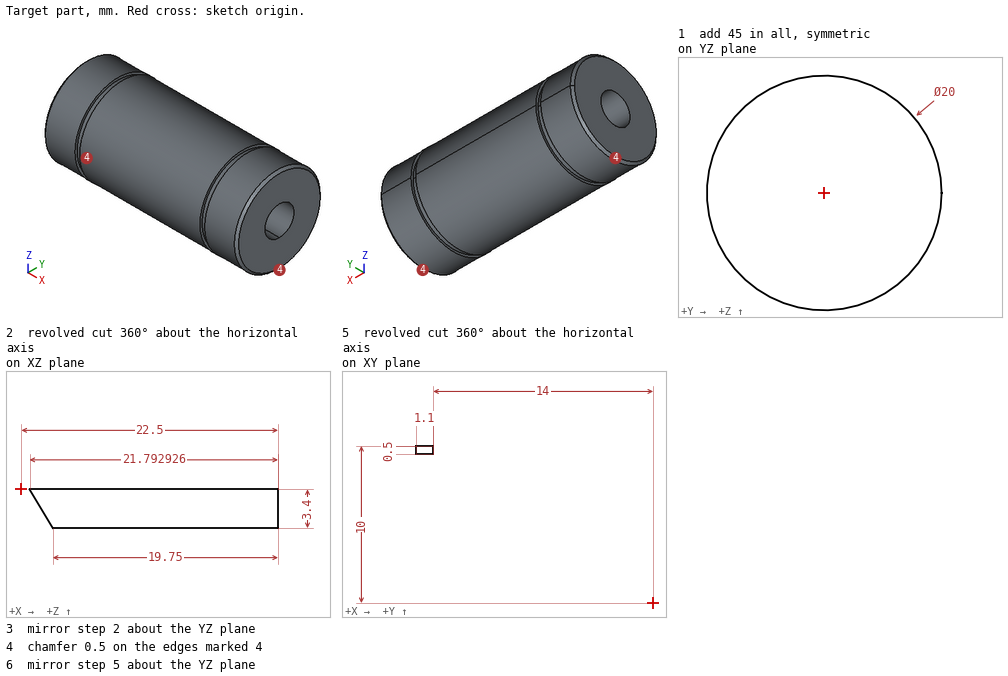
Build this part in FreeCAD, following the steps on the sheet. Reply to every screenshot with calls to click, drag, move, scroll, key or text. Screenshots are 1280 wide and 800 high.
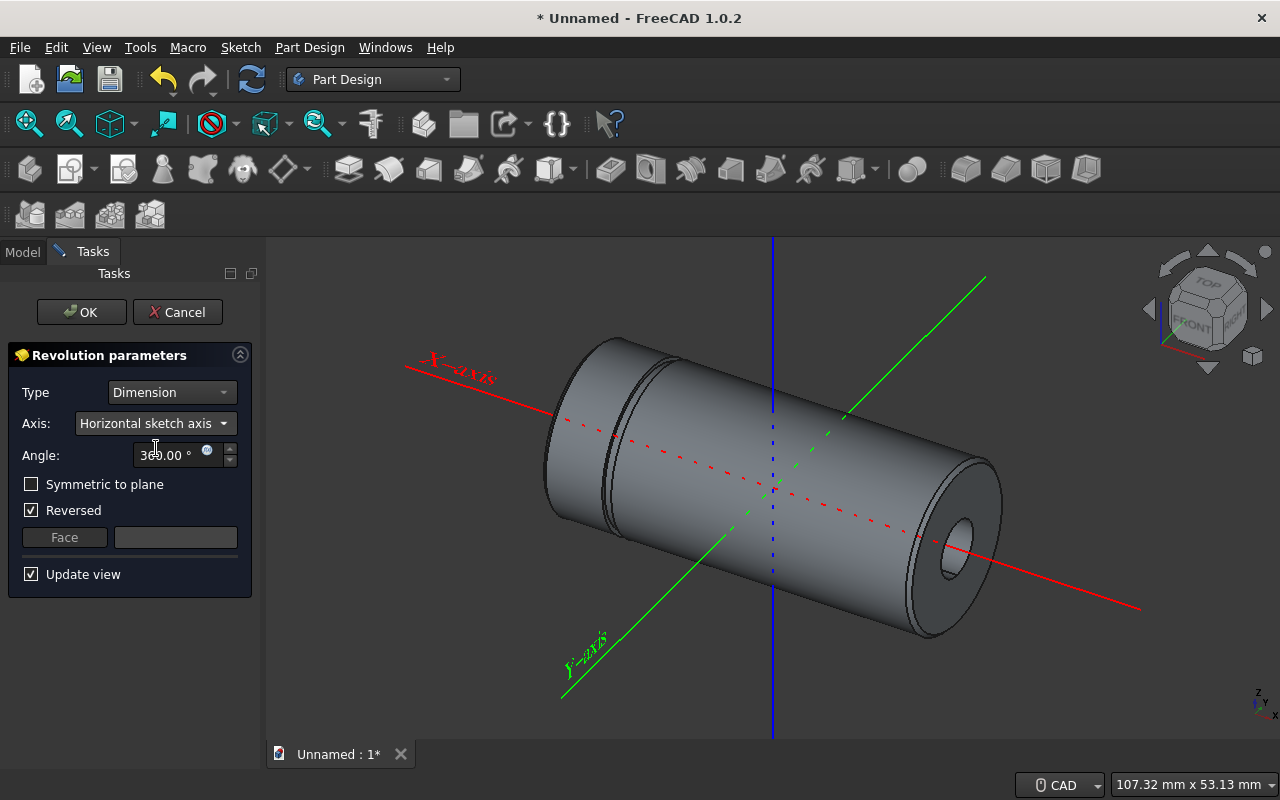
click(82, 312)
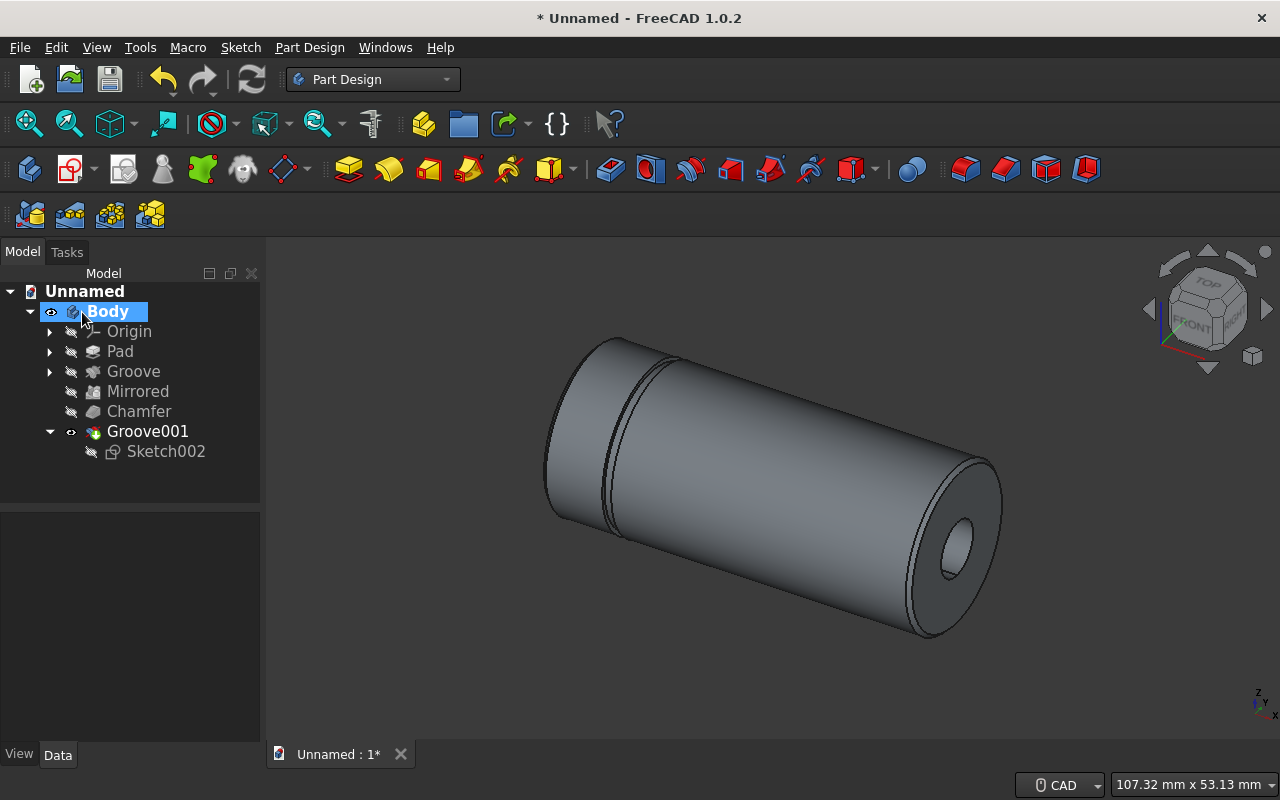
click(116, 432)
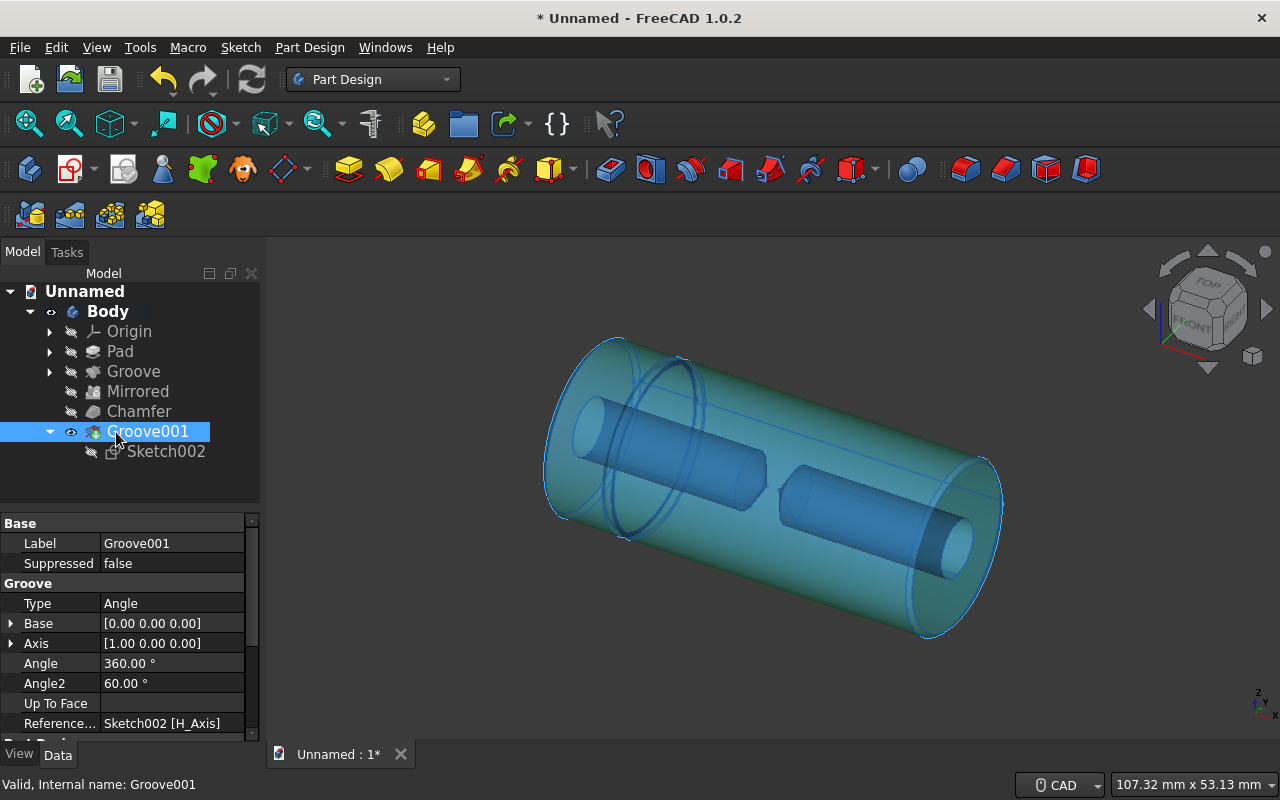
click(30, 214)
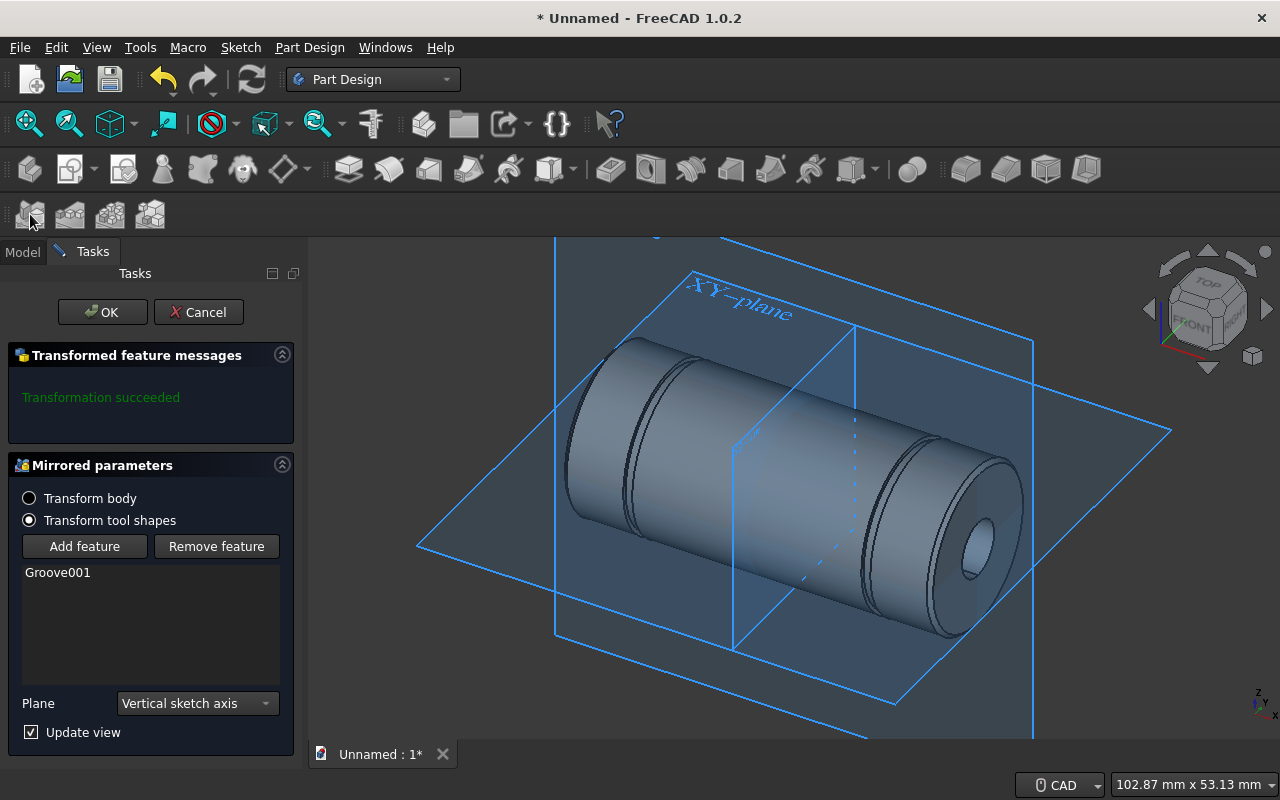
click(198, 704)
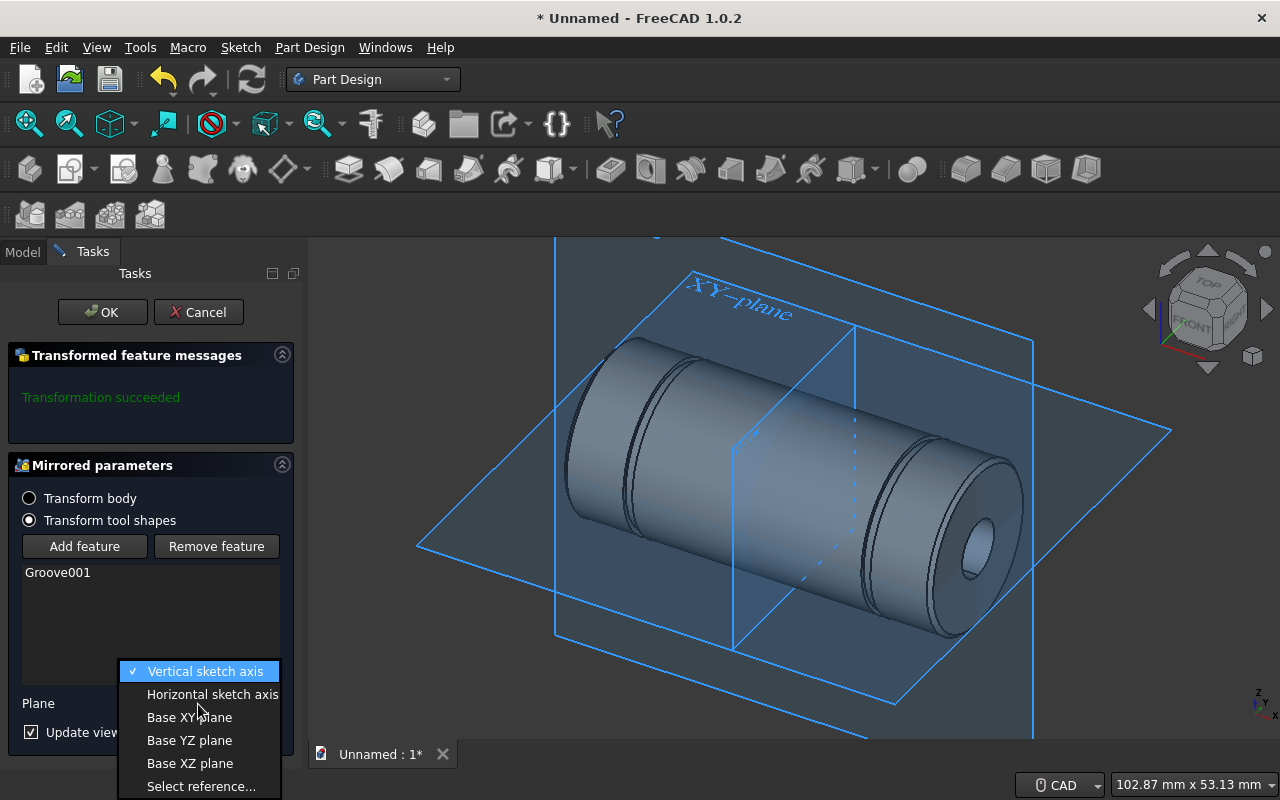
click(198, 740)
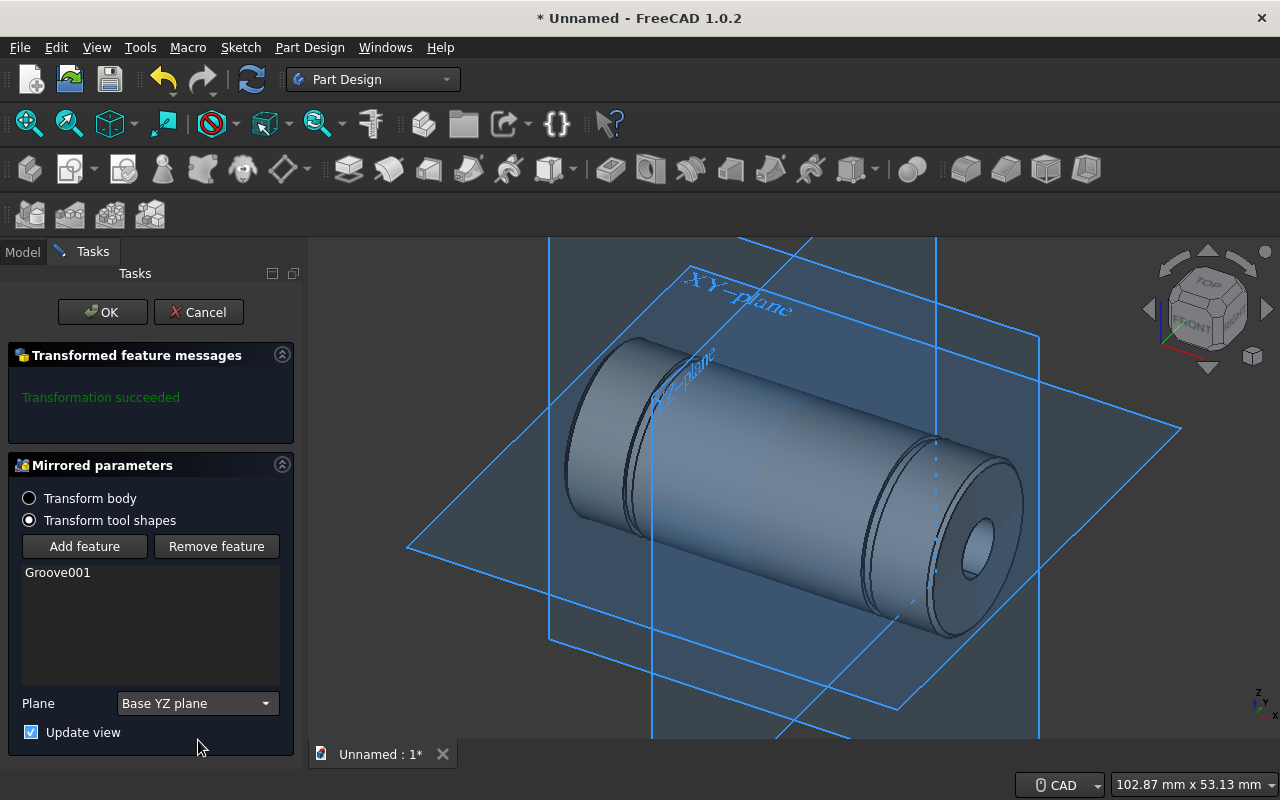
click(103, 312)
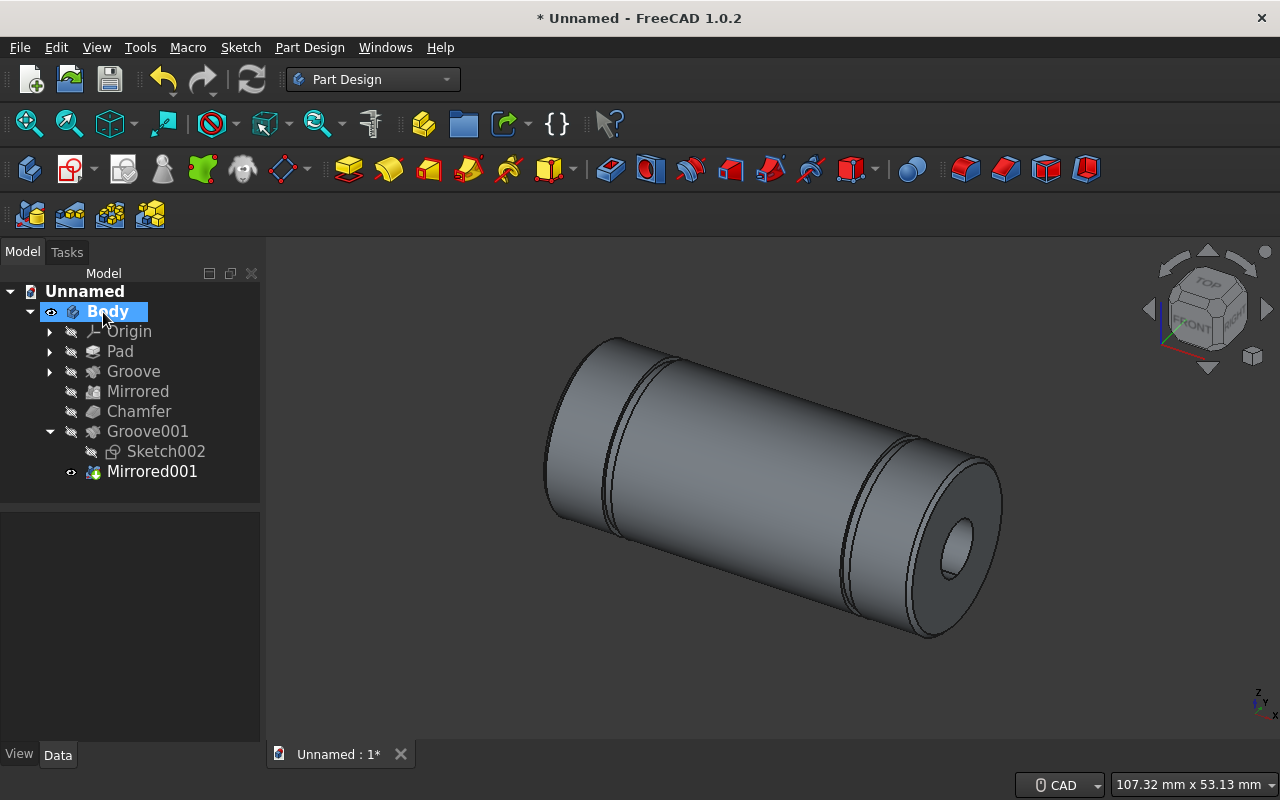
key(0)